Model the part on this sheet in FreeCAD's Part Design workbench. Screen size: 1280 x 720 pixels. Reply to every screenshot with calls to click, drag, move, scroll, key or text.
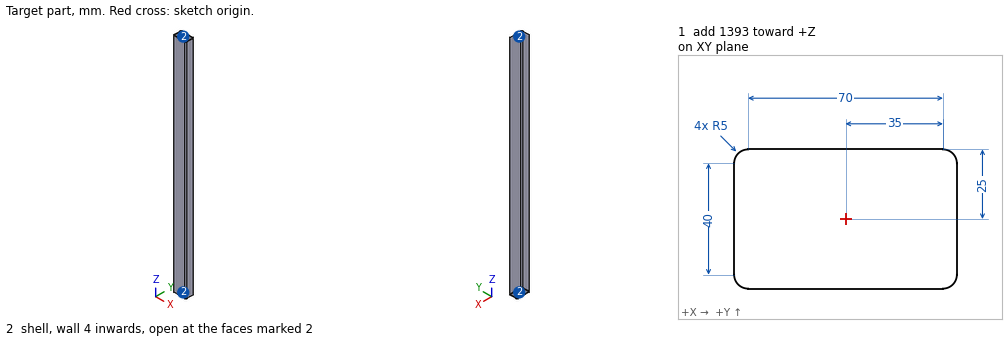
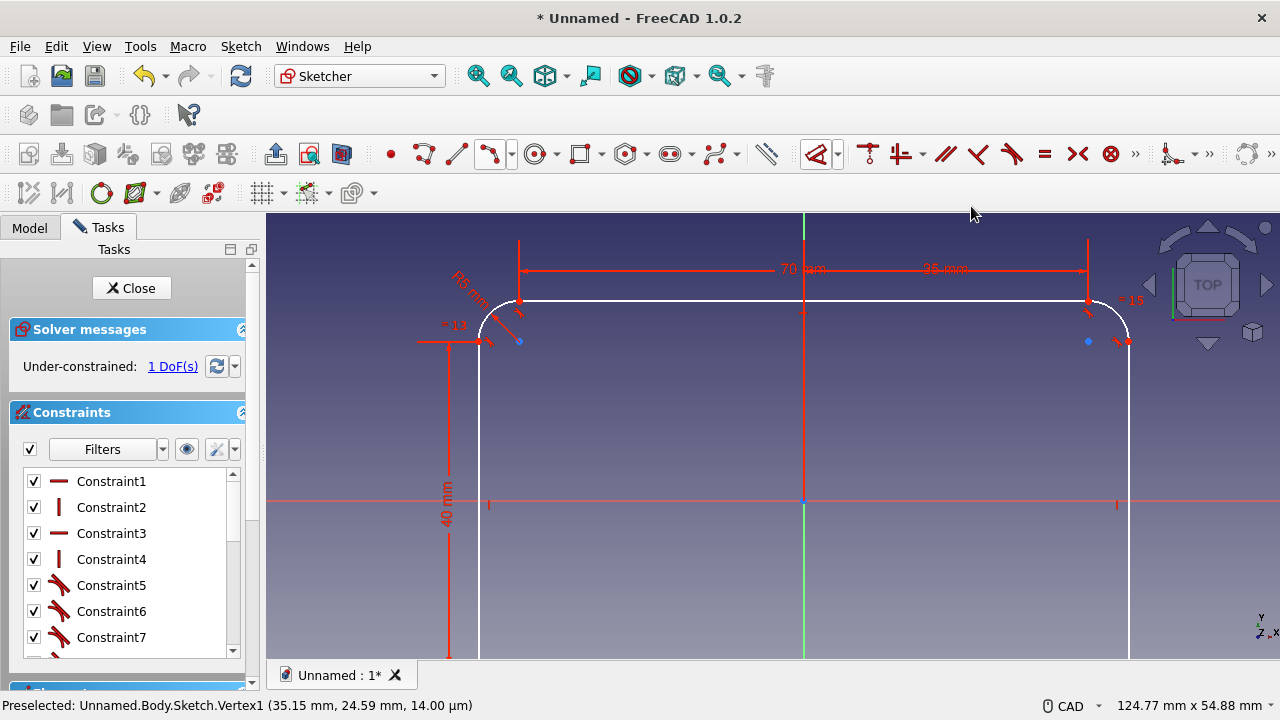
click(1088, 301)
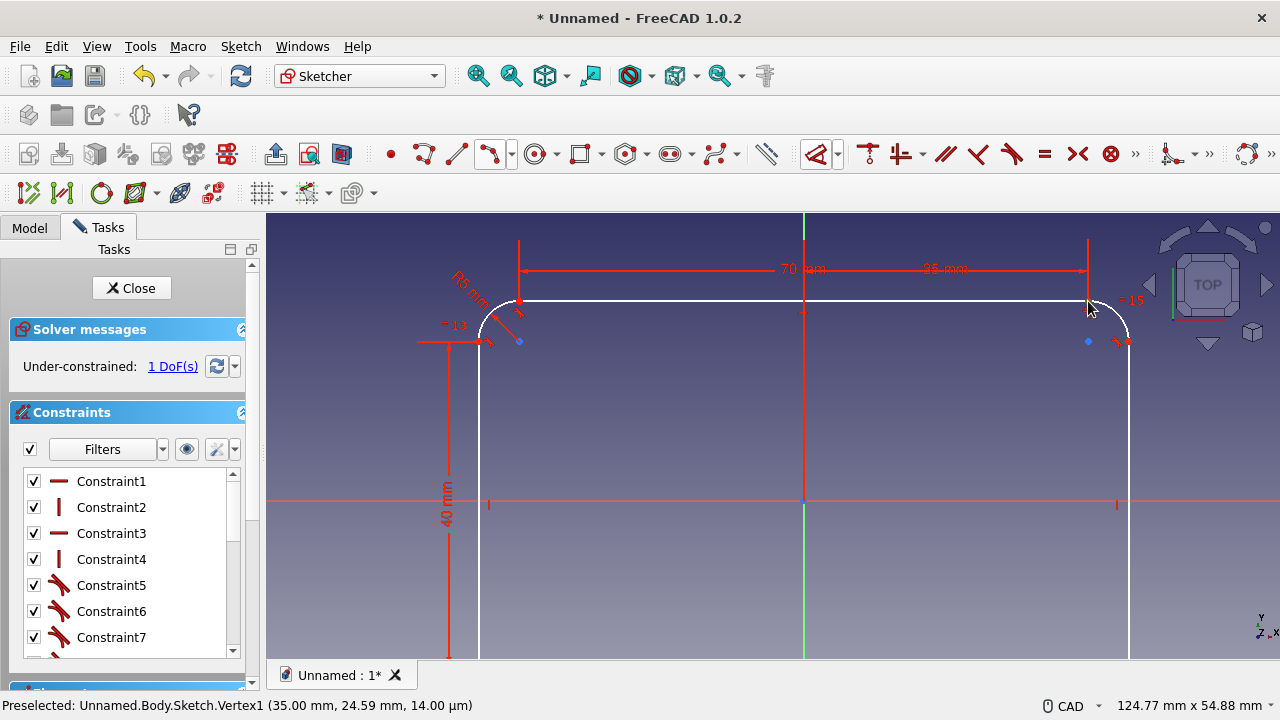
key(i)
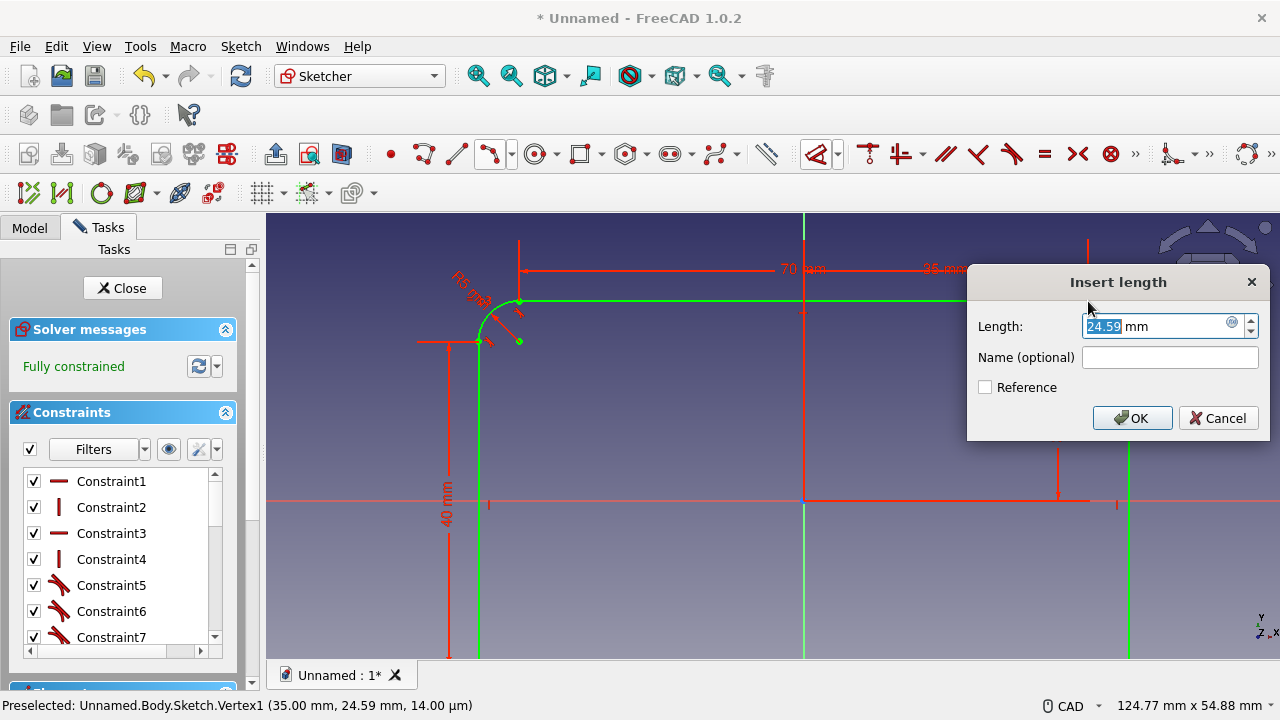
text(25)
key(Return)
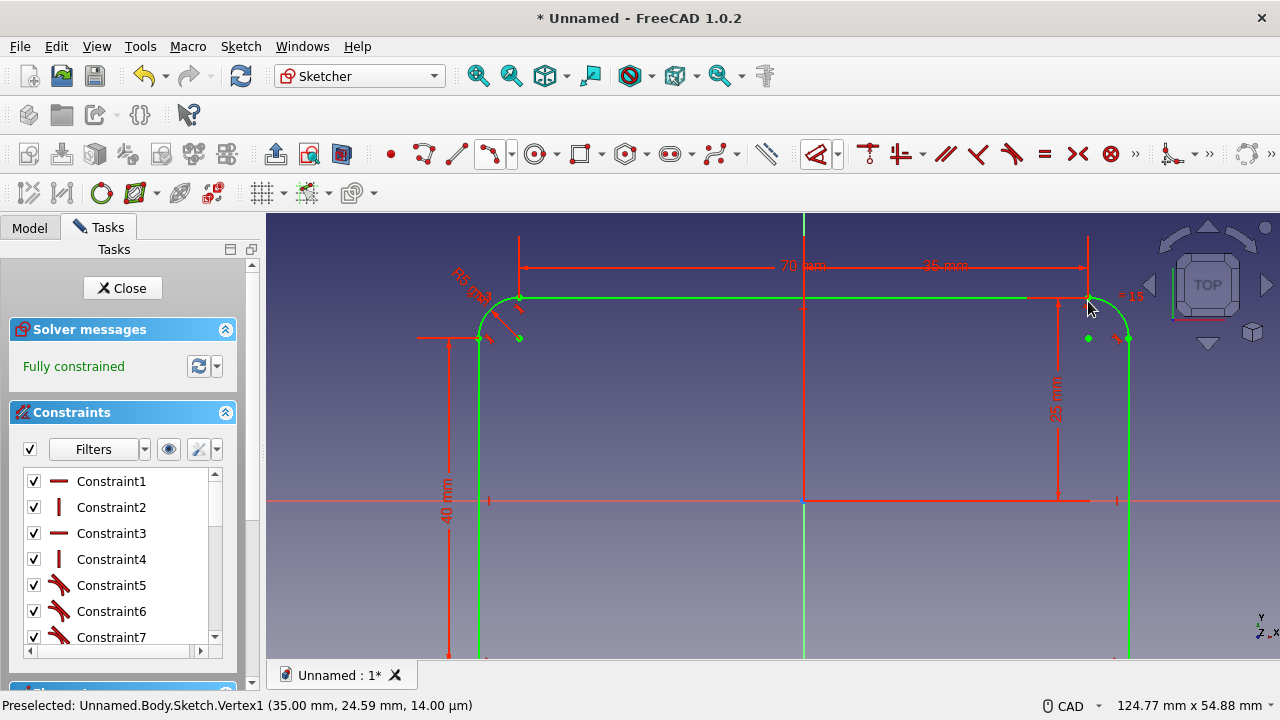
click(123, 288)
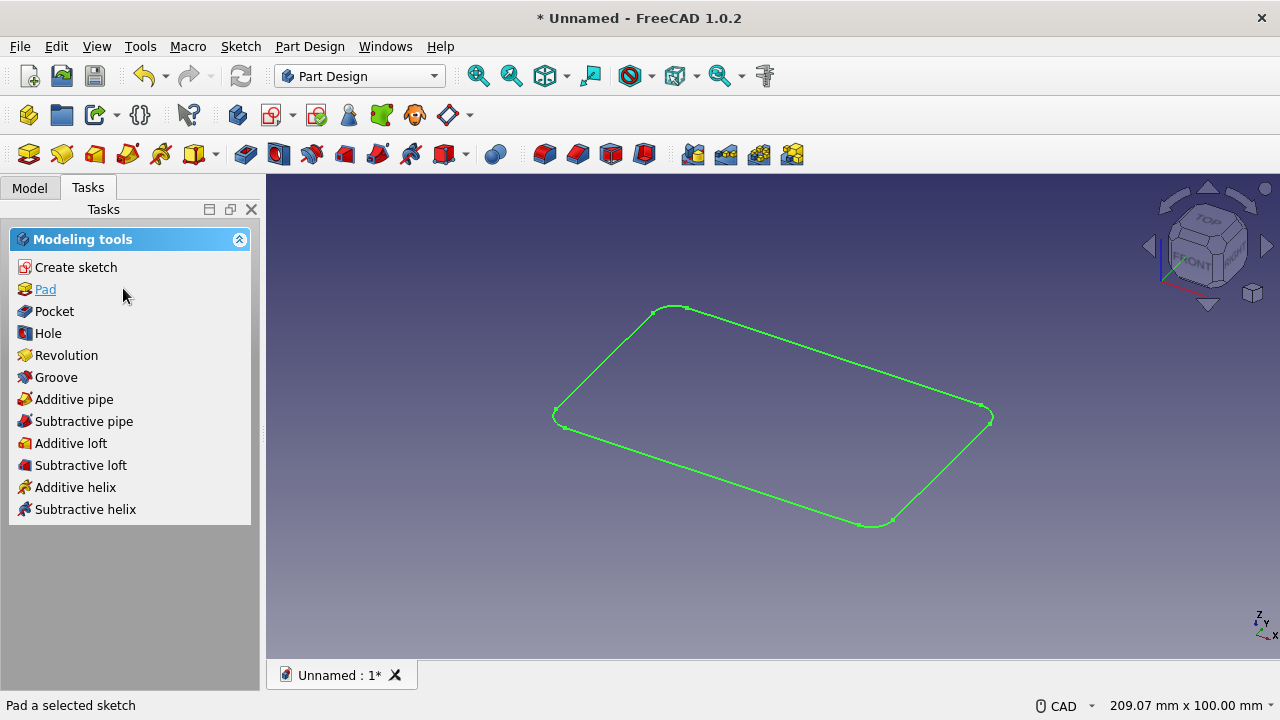
click(29, 154)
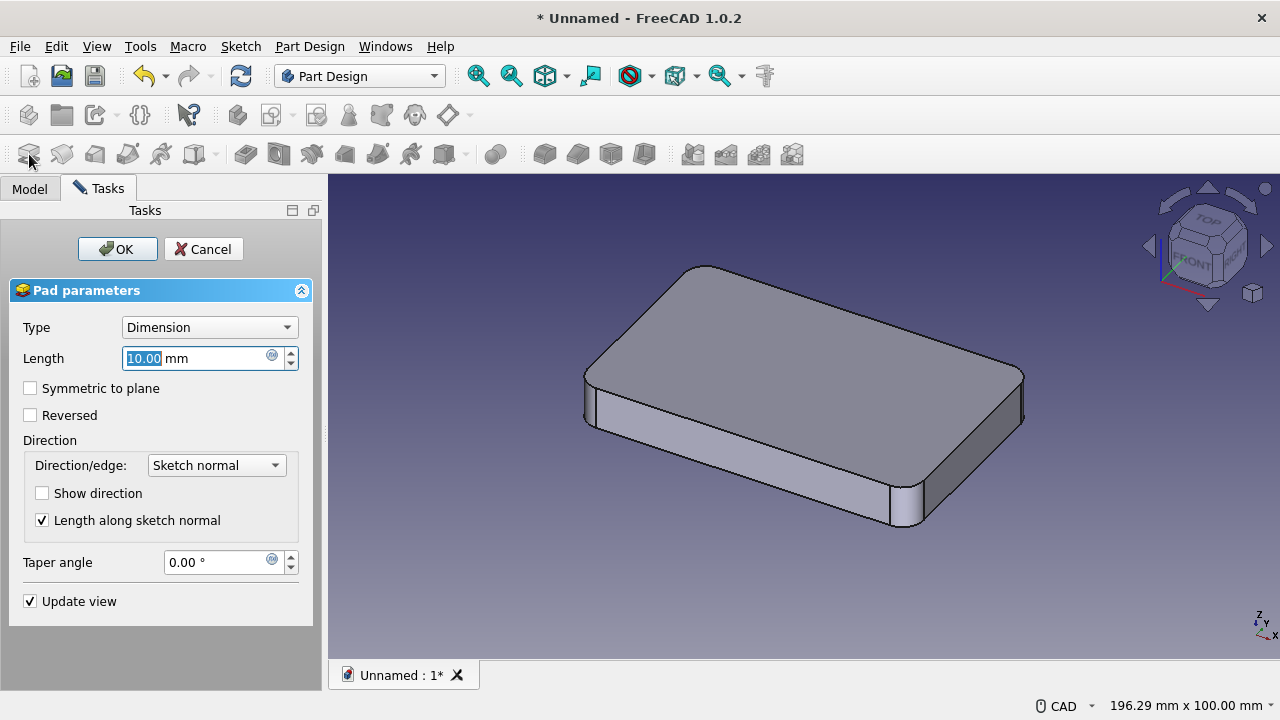
text(1393)
key(Tab)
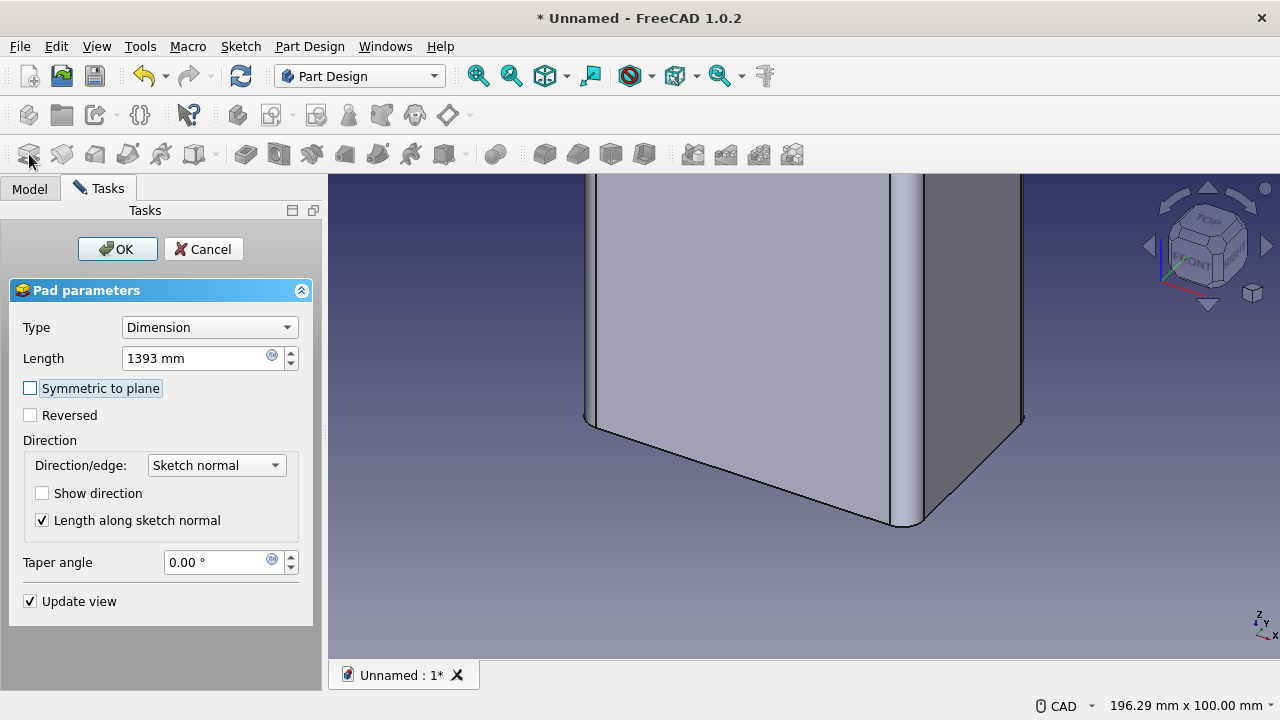
click(118, 249)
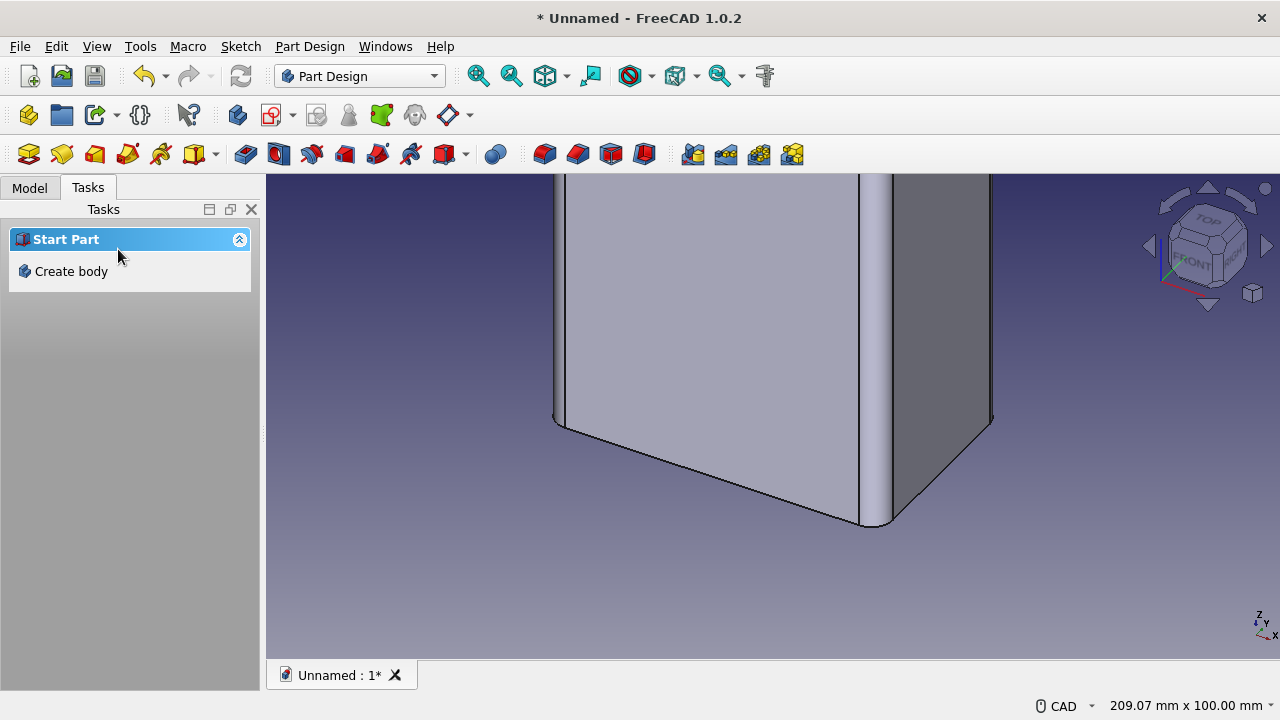
click(479, 76)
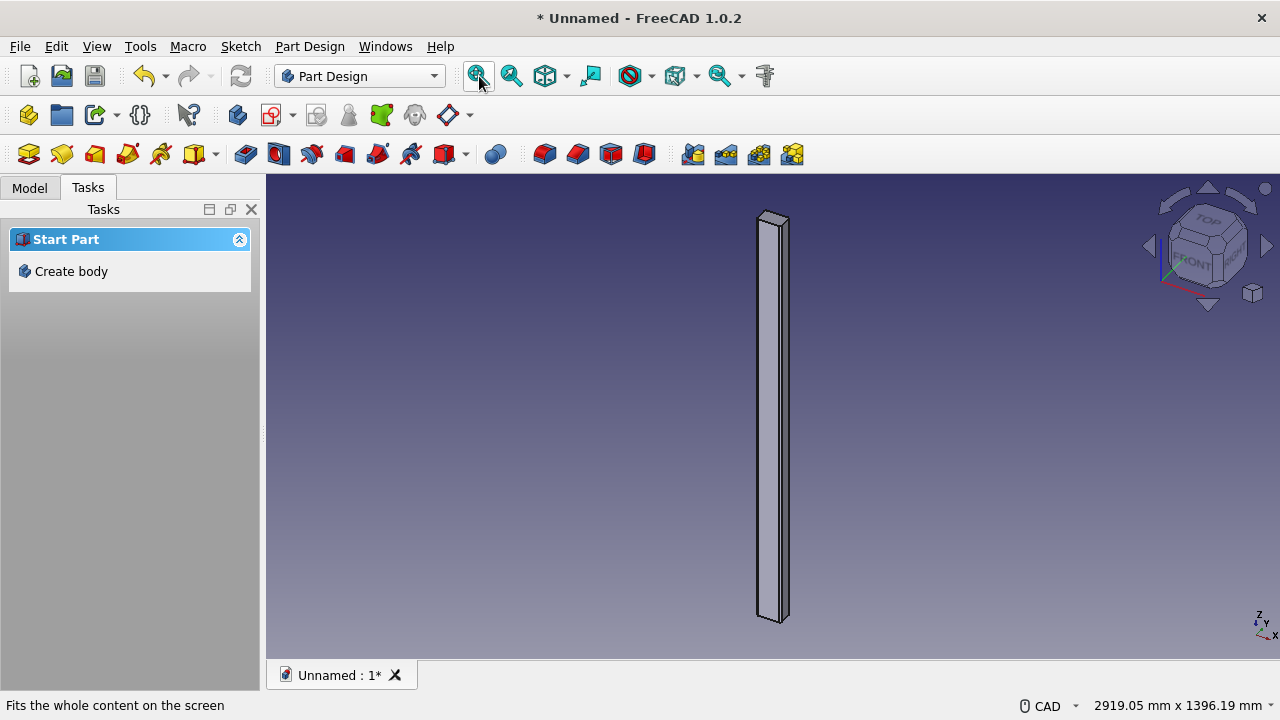
key(0)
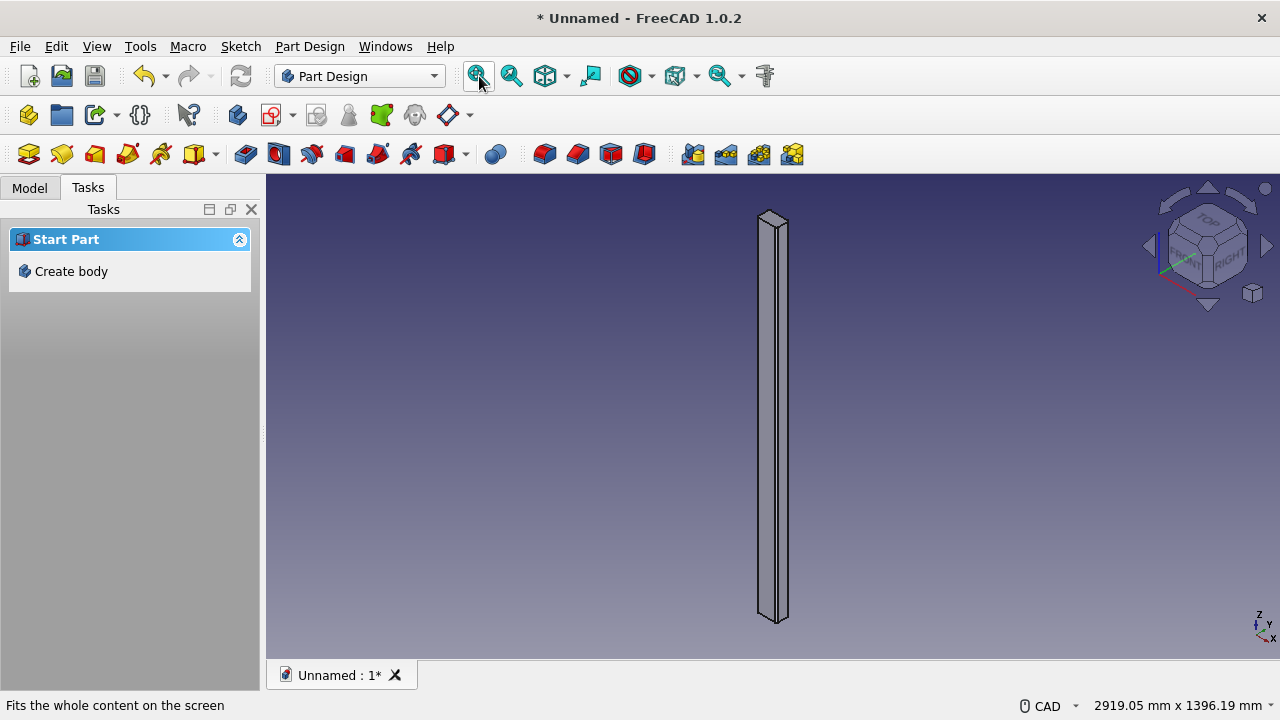
key(2)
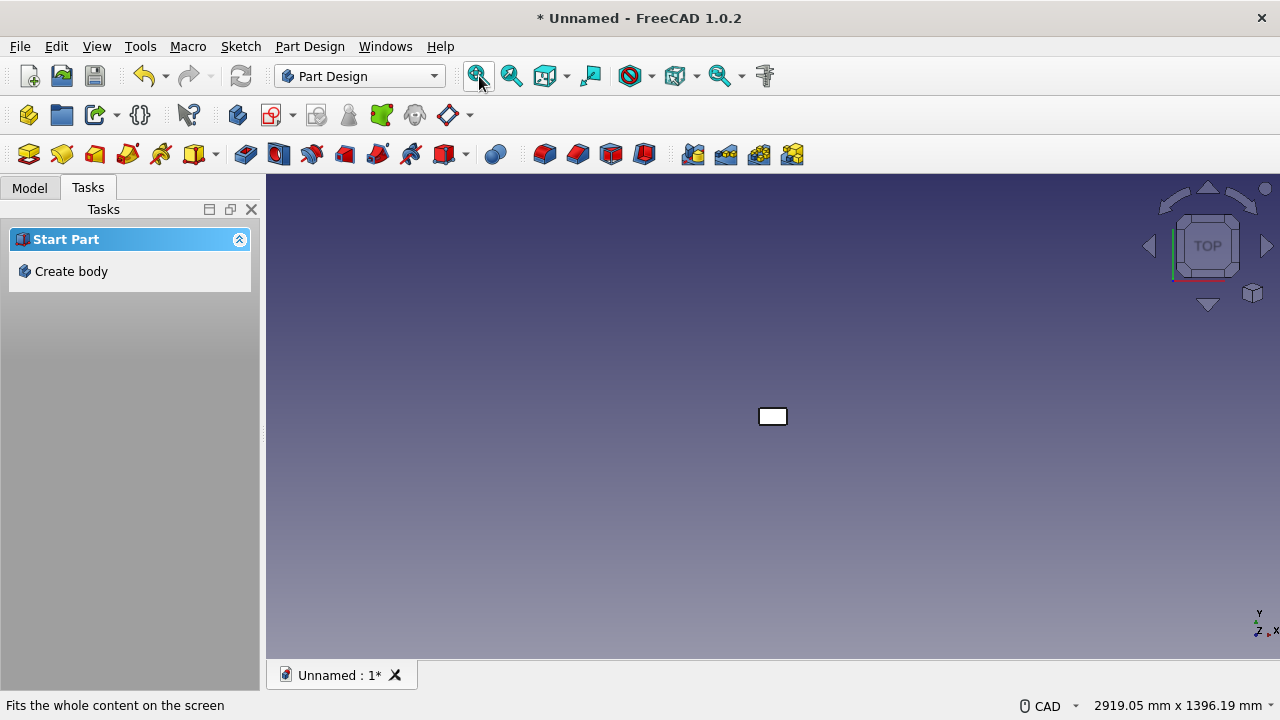
click(479, 76)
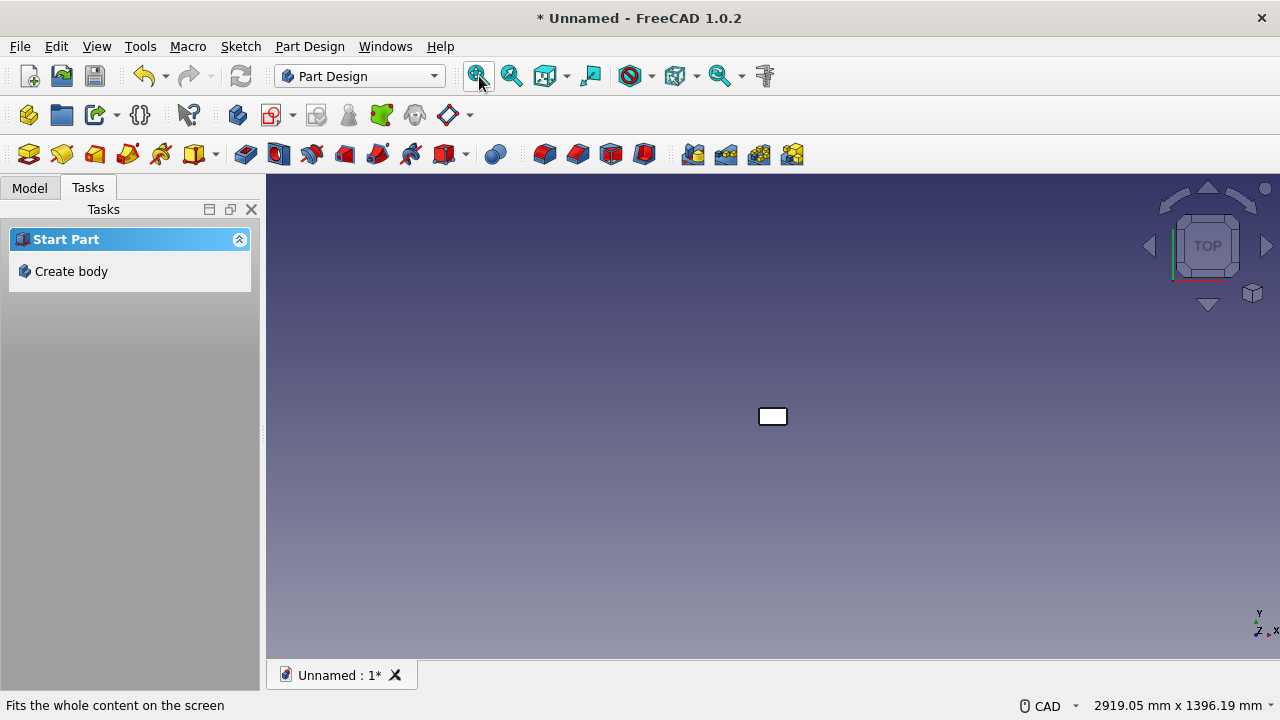
click(777, 415)